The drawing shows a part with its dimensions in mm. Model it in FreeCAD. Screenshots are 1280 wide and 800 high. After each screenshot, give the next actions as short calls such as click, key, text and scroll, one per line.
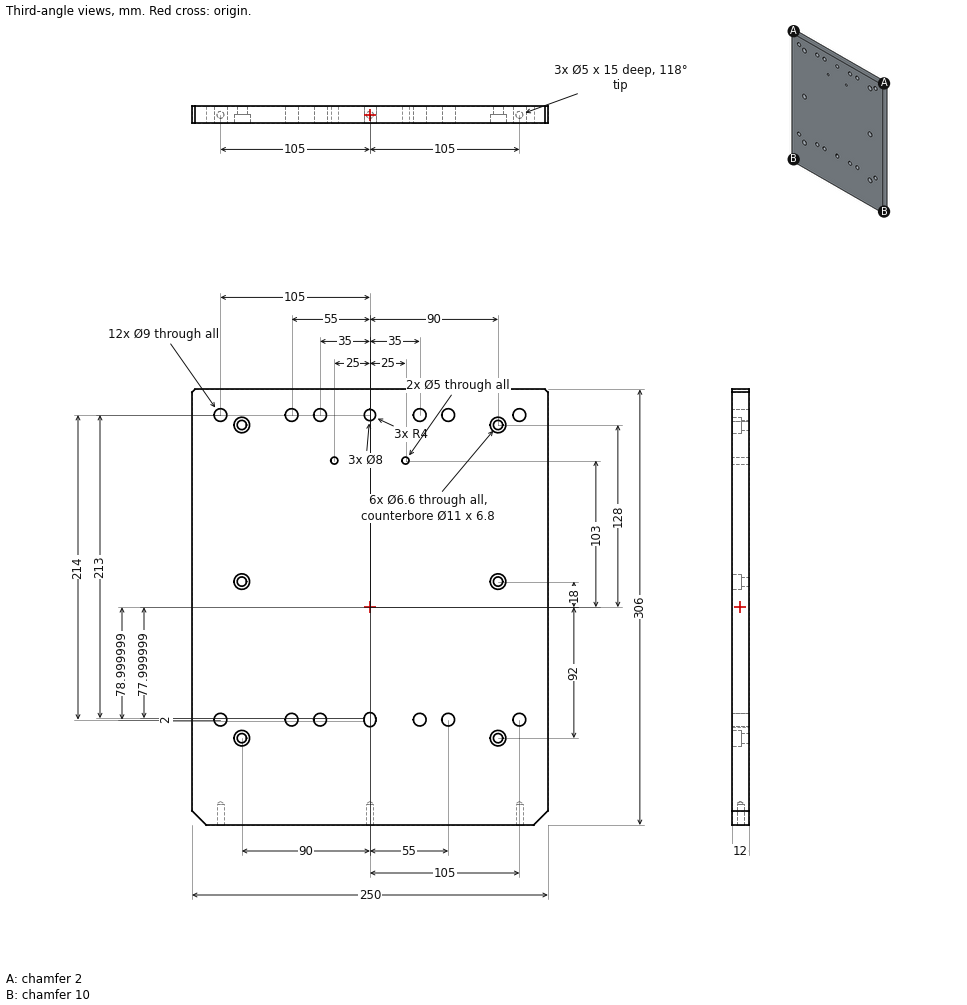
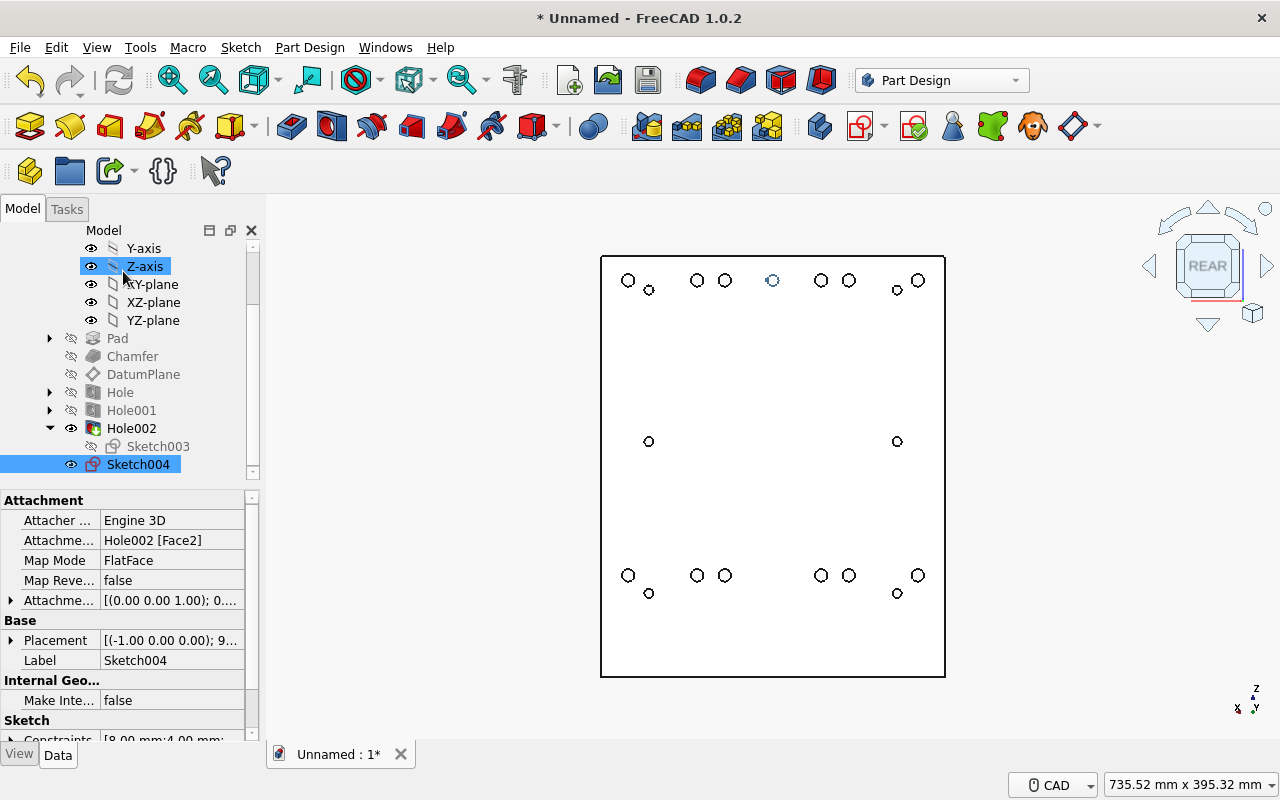
click(292, 126)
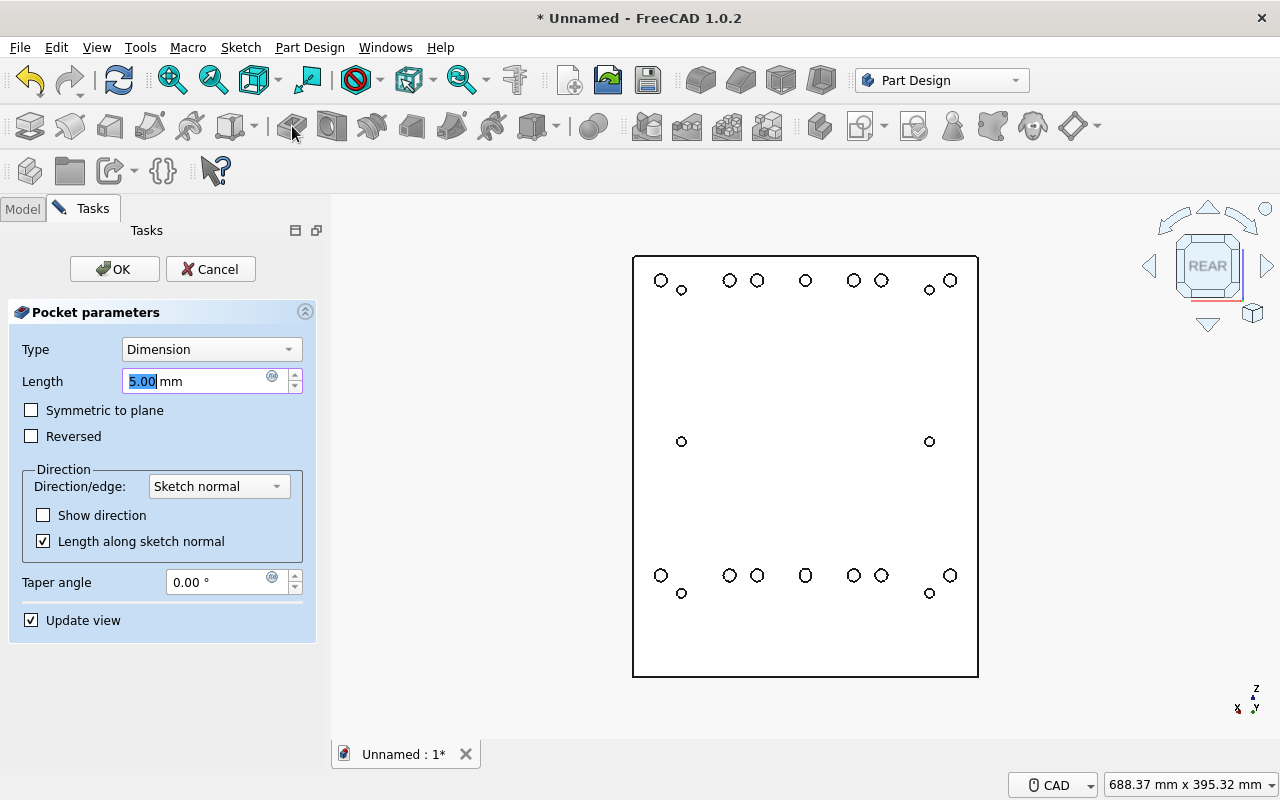
click(212, 350)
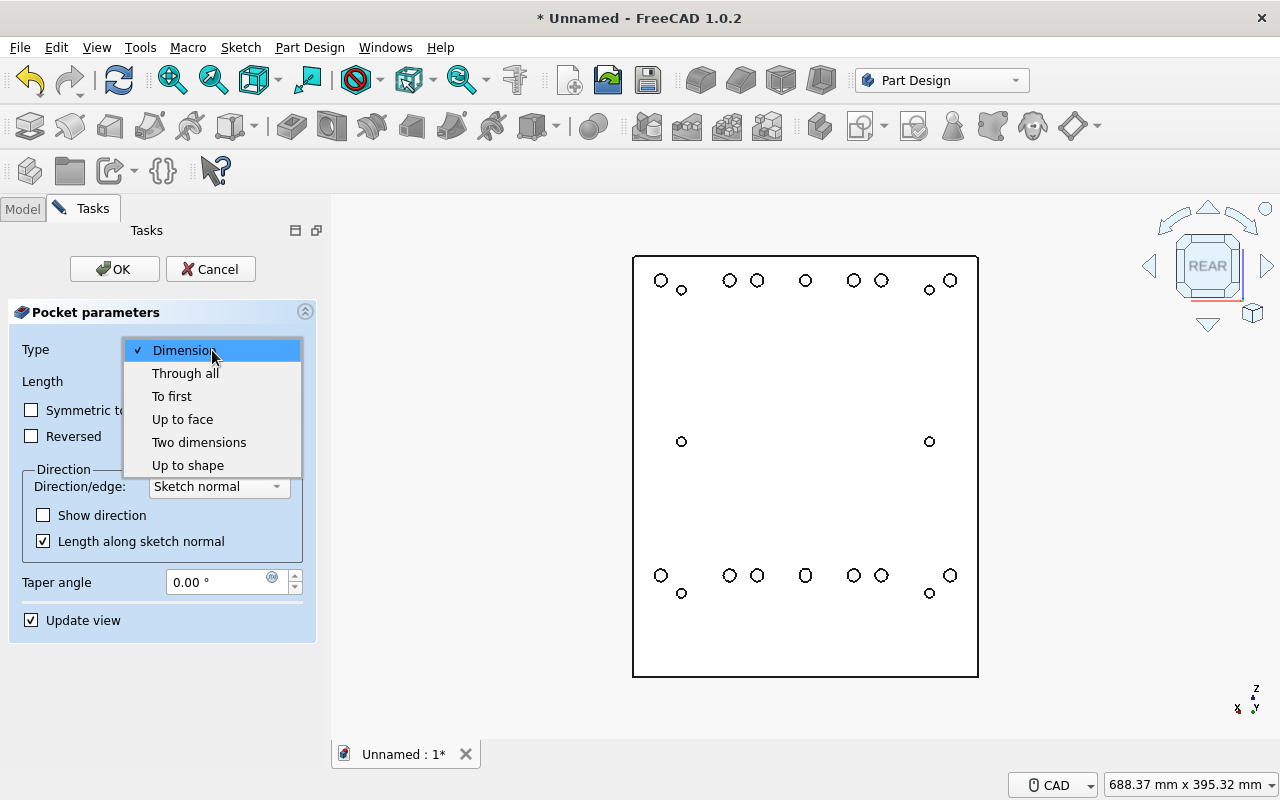
click(212, 374)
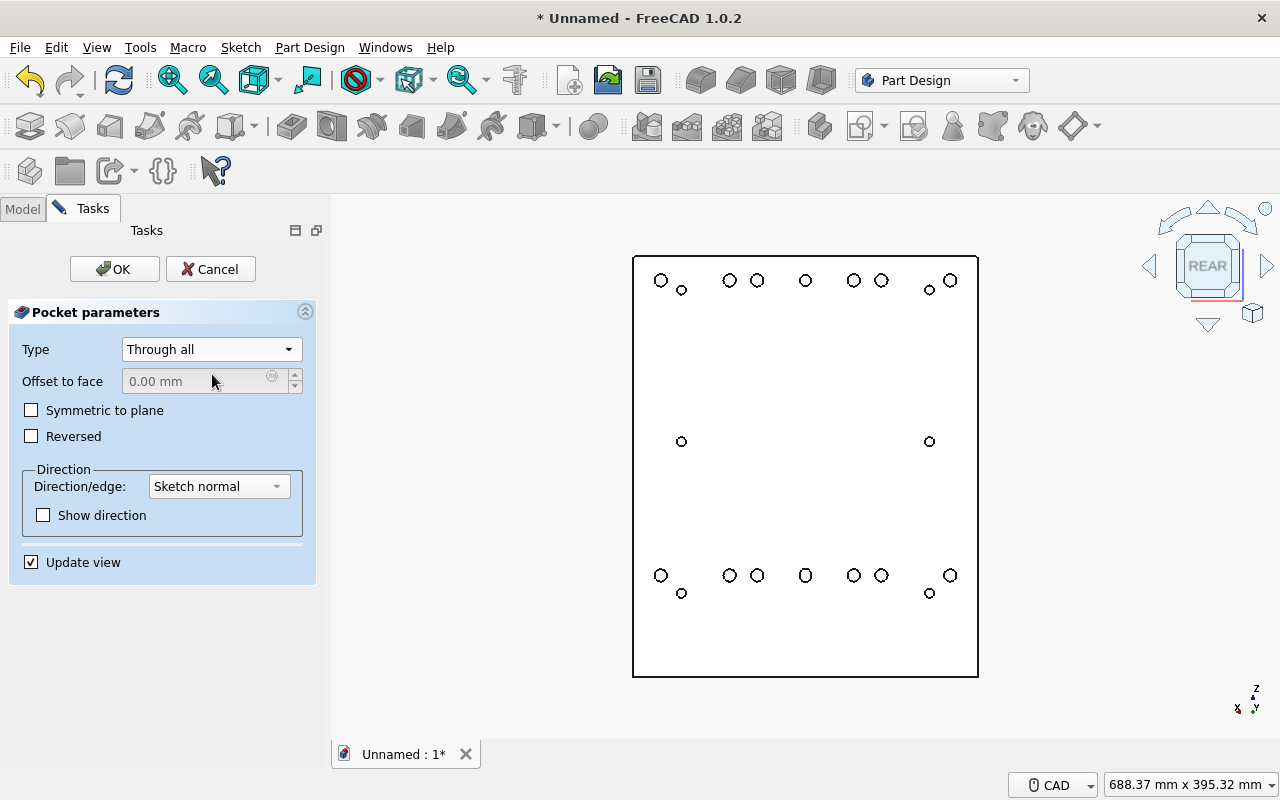
click(115, 269)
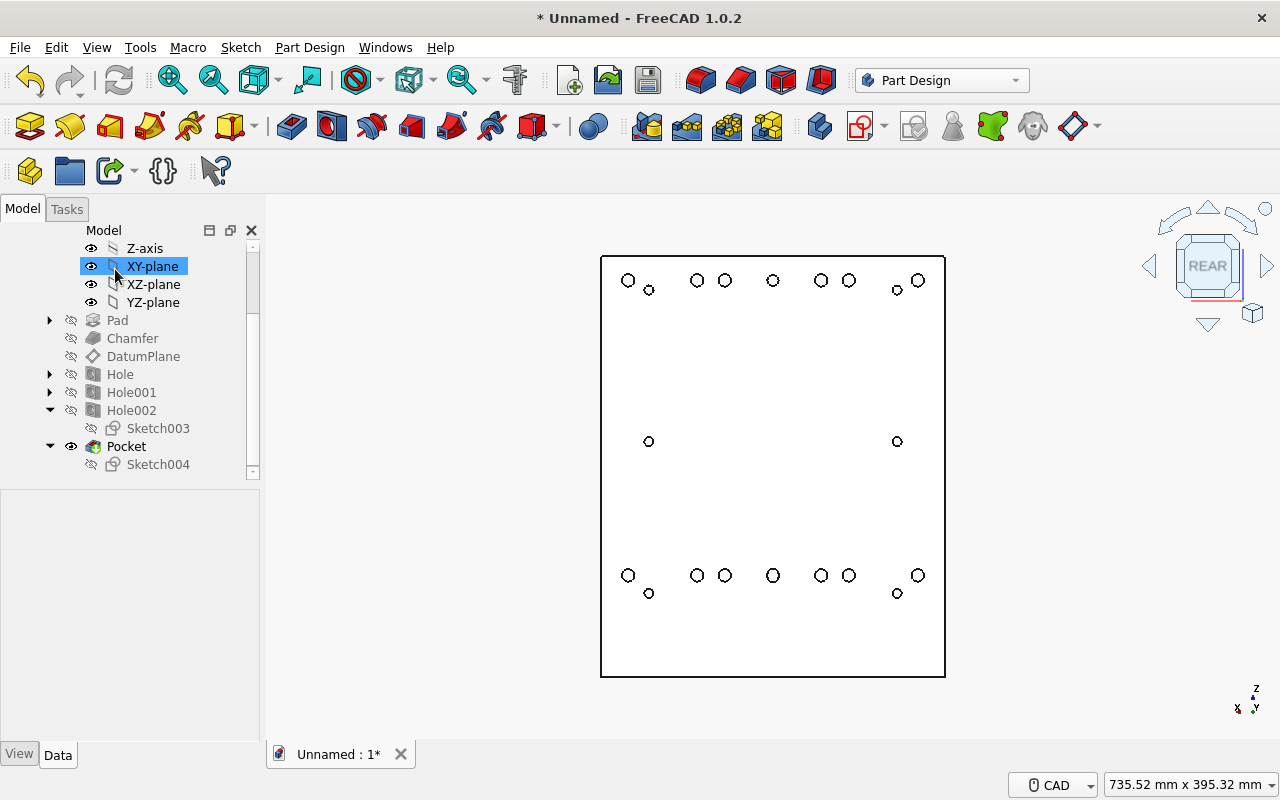
click(773, 405)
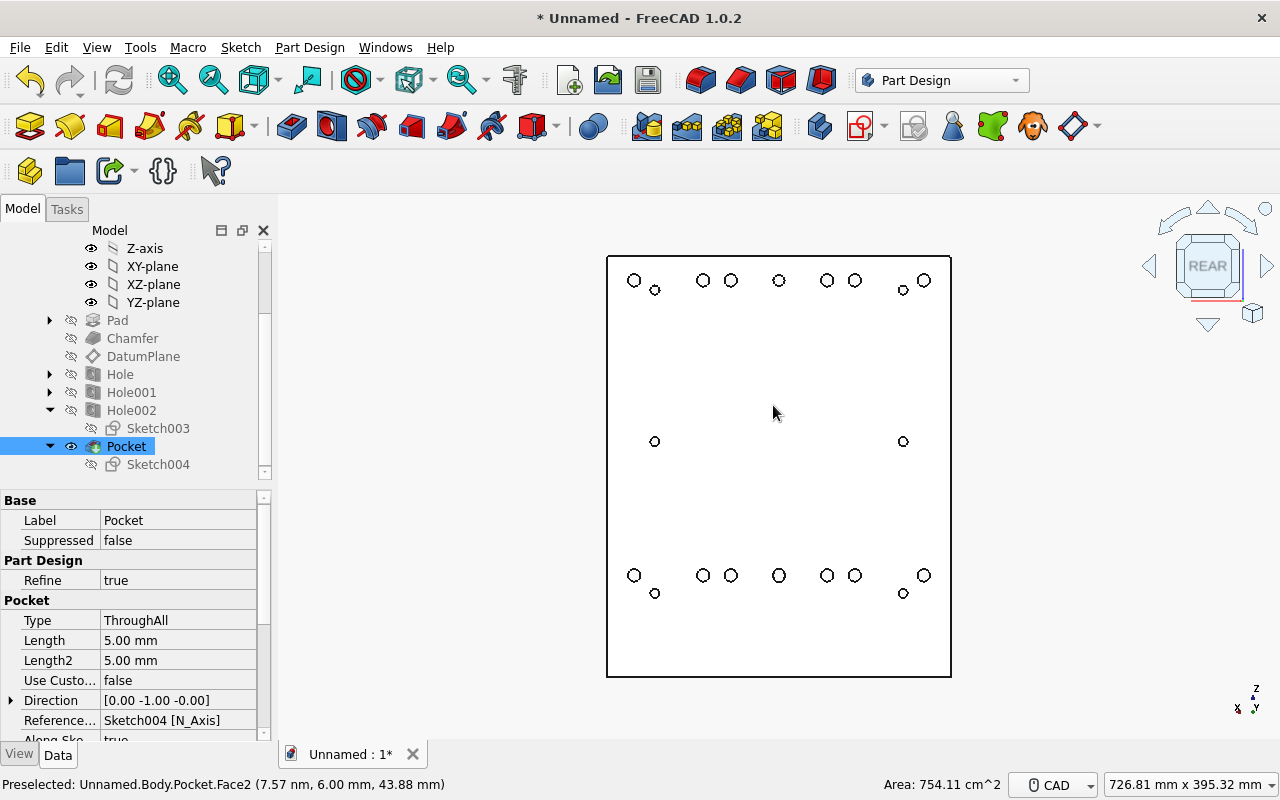
click(860, 126)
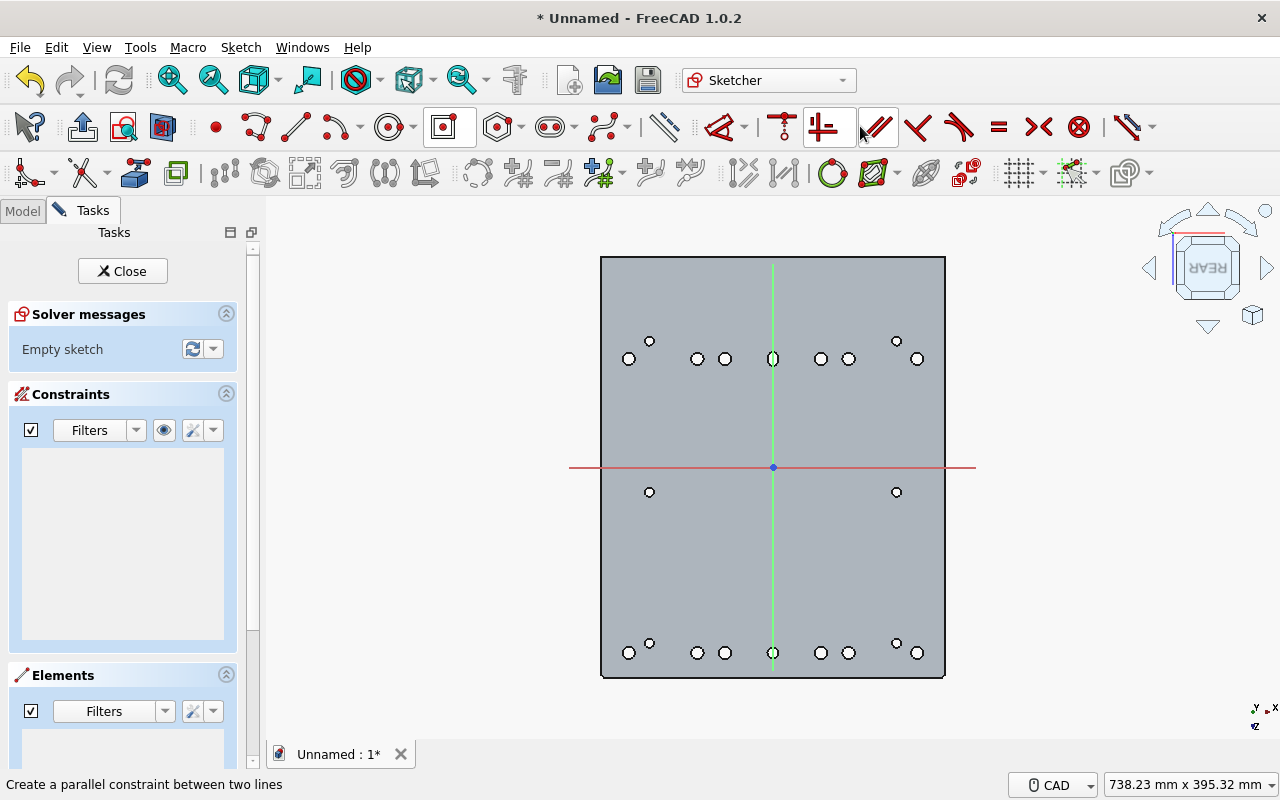
scroll(829, 599, up, 4)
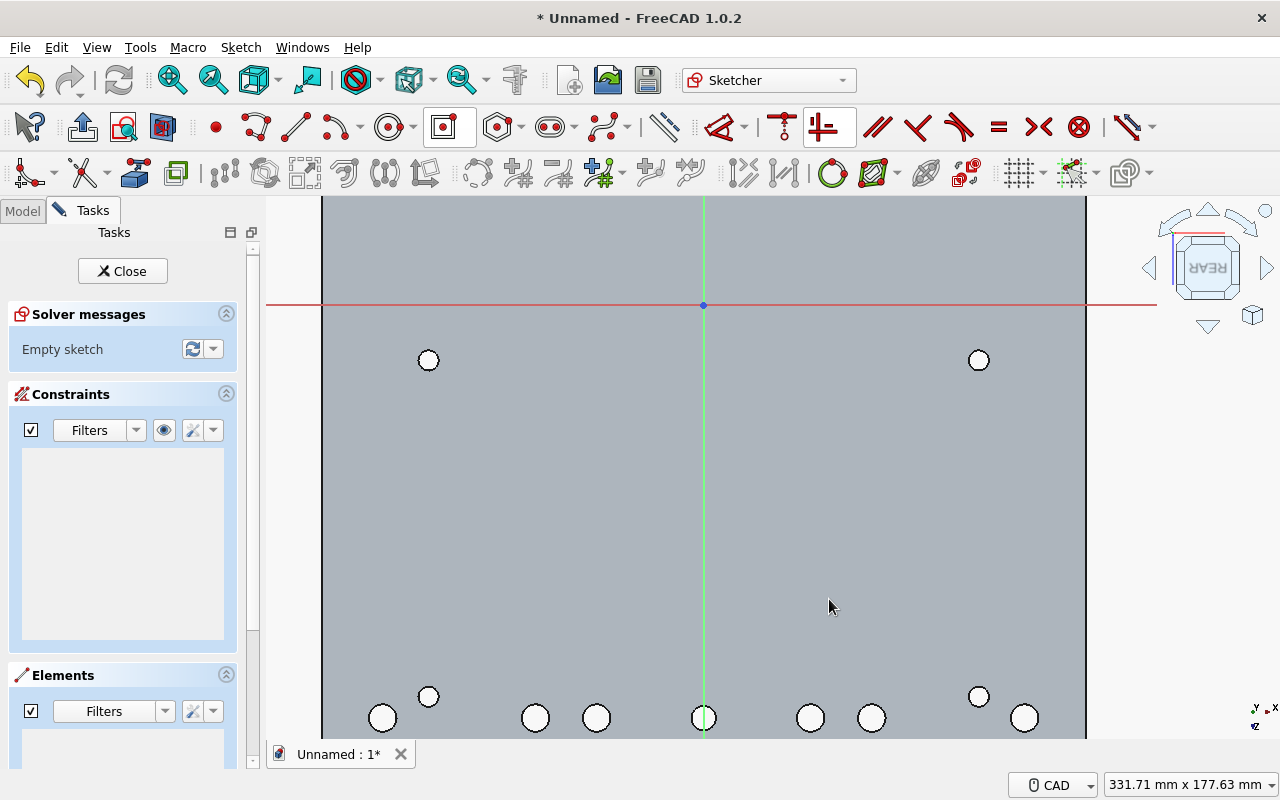
click(390, 128)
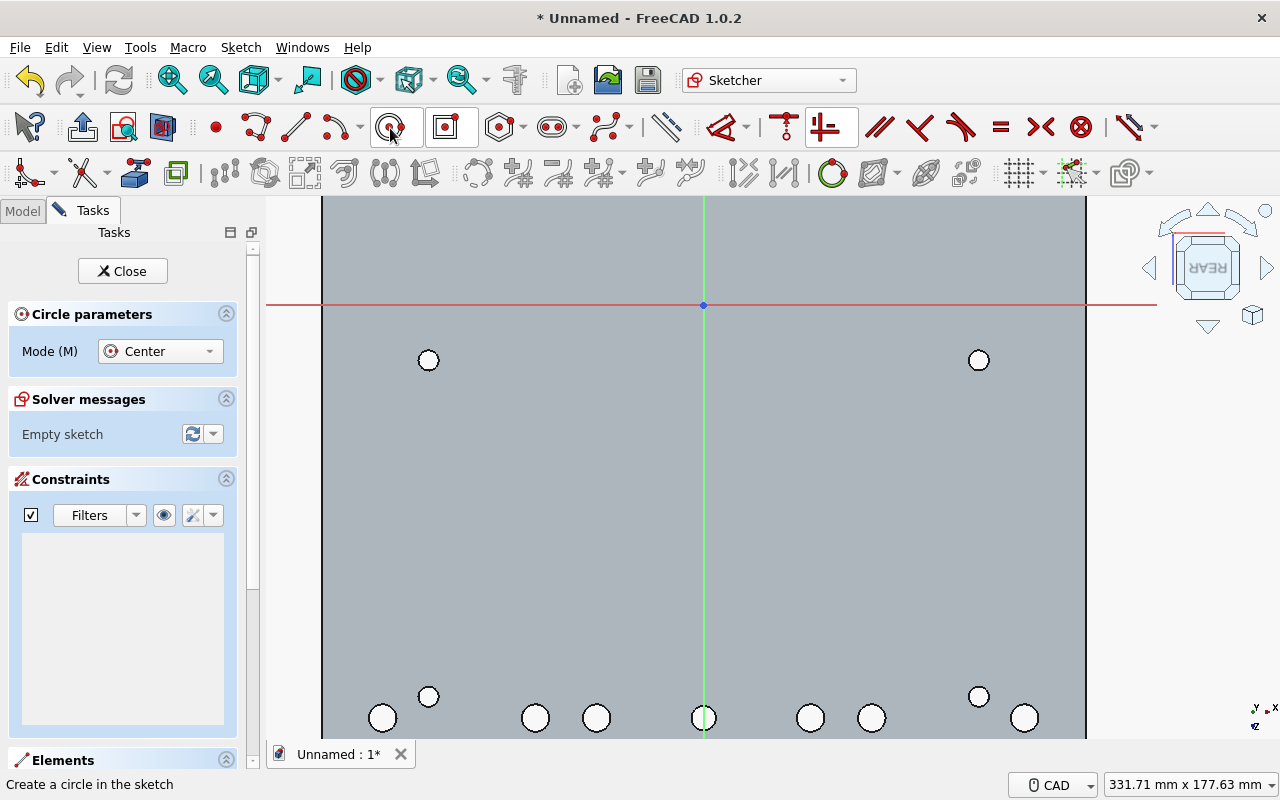
scroll(780, 620, up, 6)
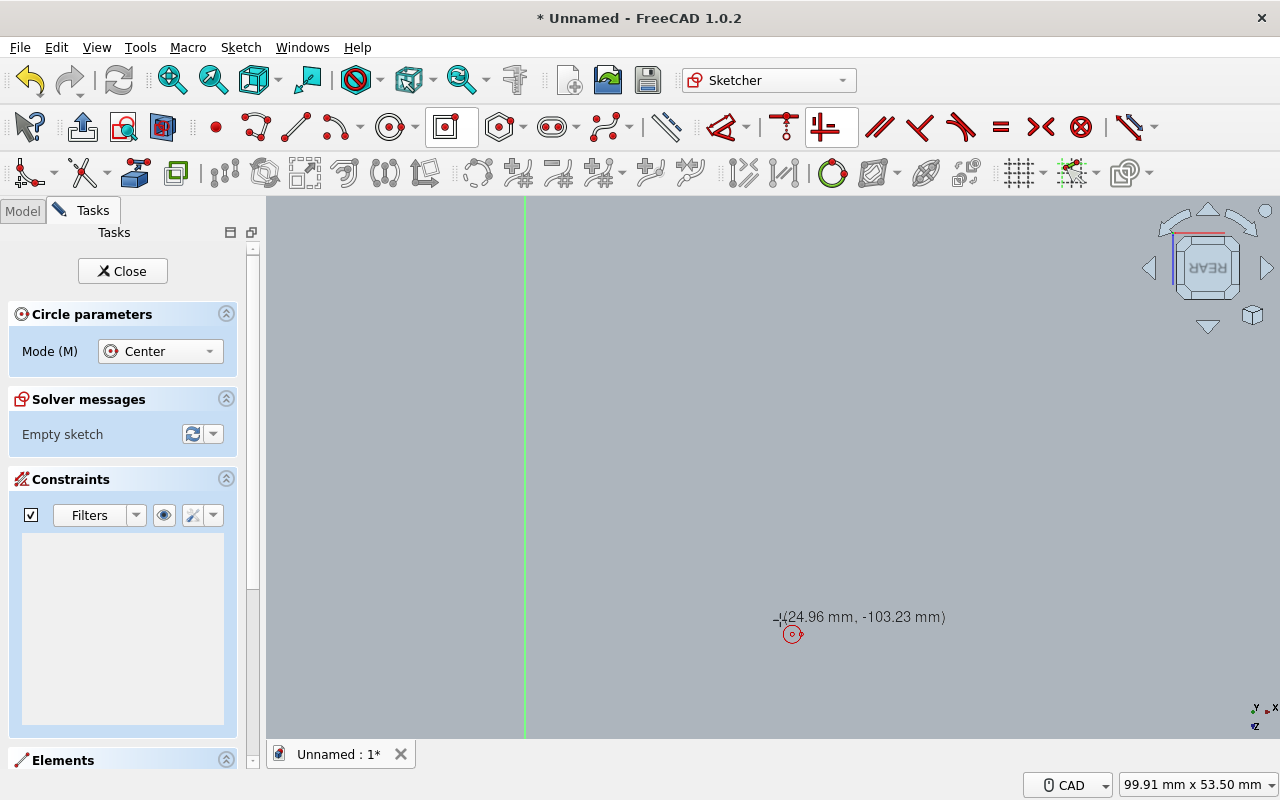
click(779, 619)
move(797, 601)